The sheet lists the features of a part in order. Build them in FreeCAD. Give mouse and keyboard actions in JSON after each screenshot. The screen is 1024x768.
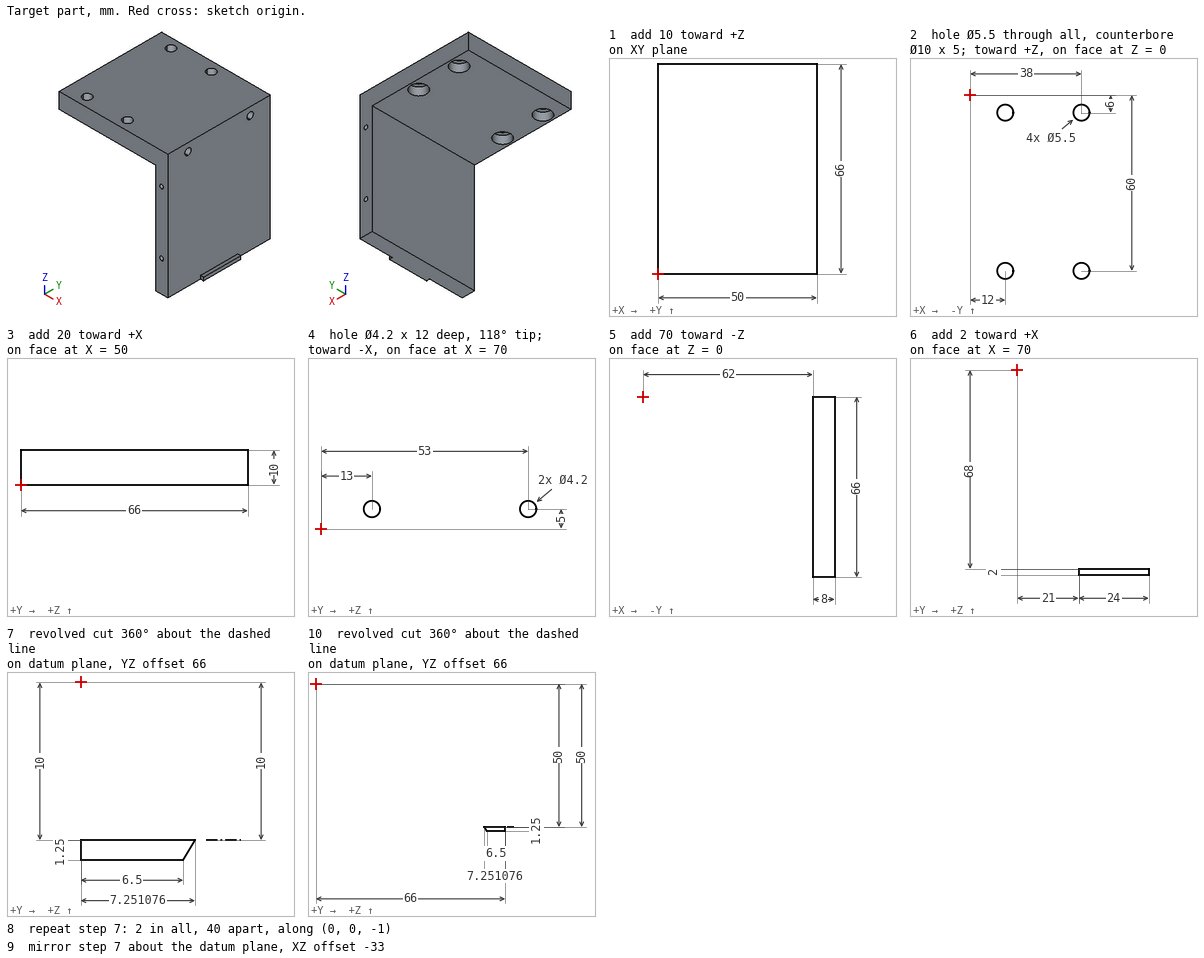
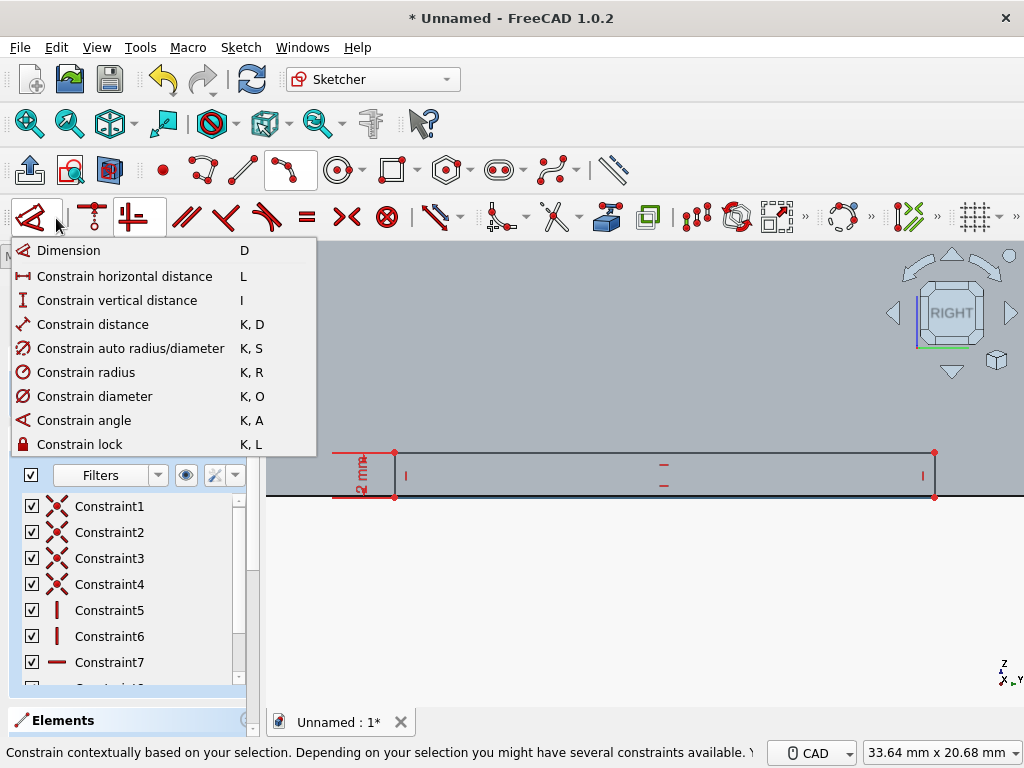
{"action": "left_click", "coordinate": [164, 276]}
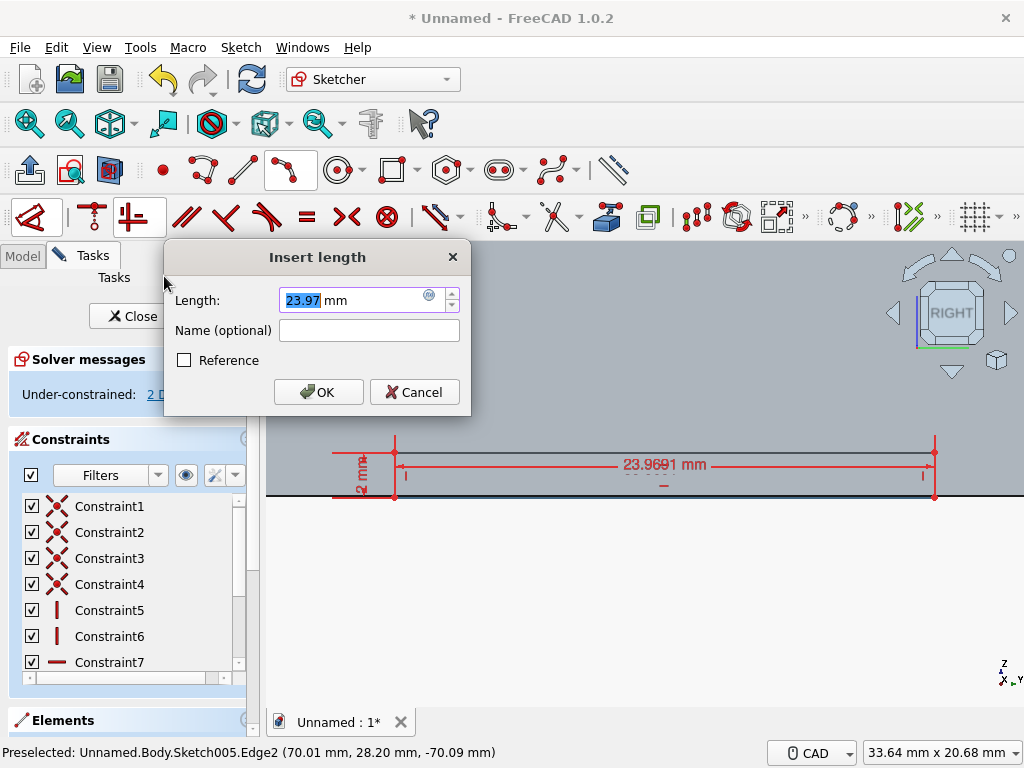
{"action": "type", "text": "24"}
{"action": "key", "text": "Return"}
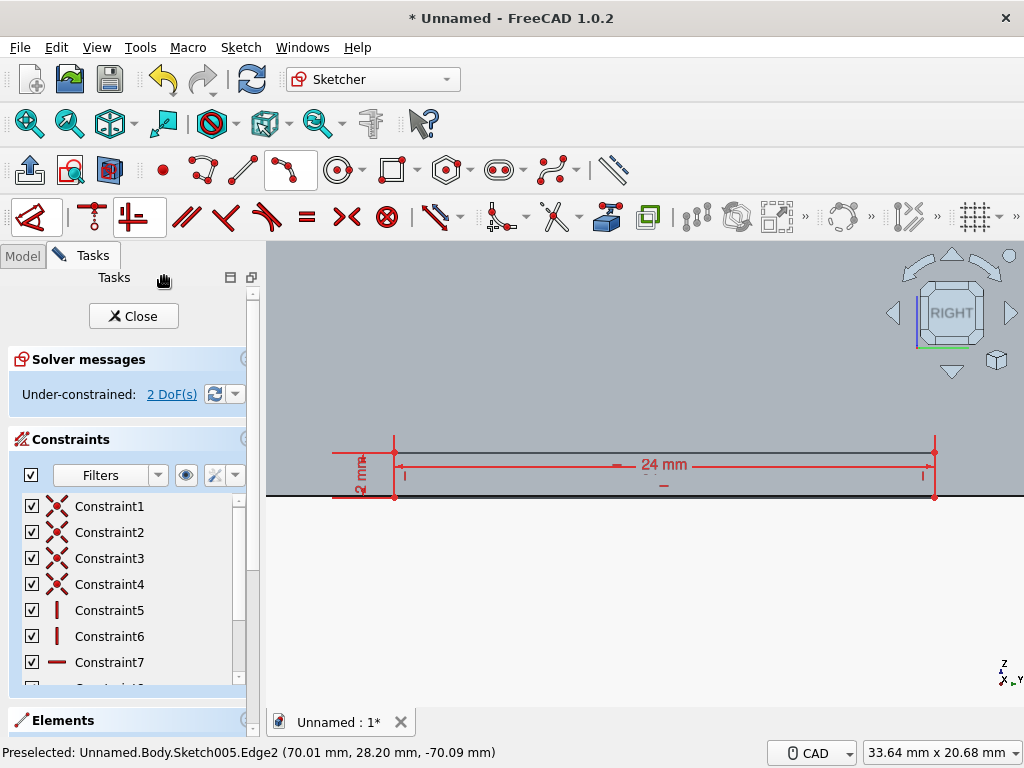
{"action": "left_click", "coordinate": [394, 453]}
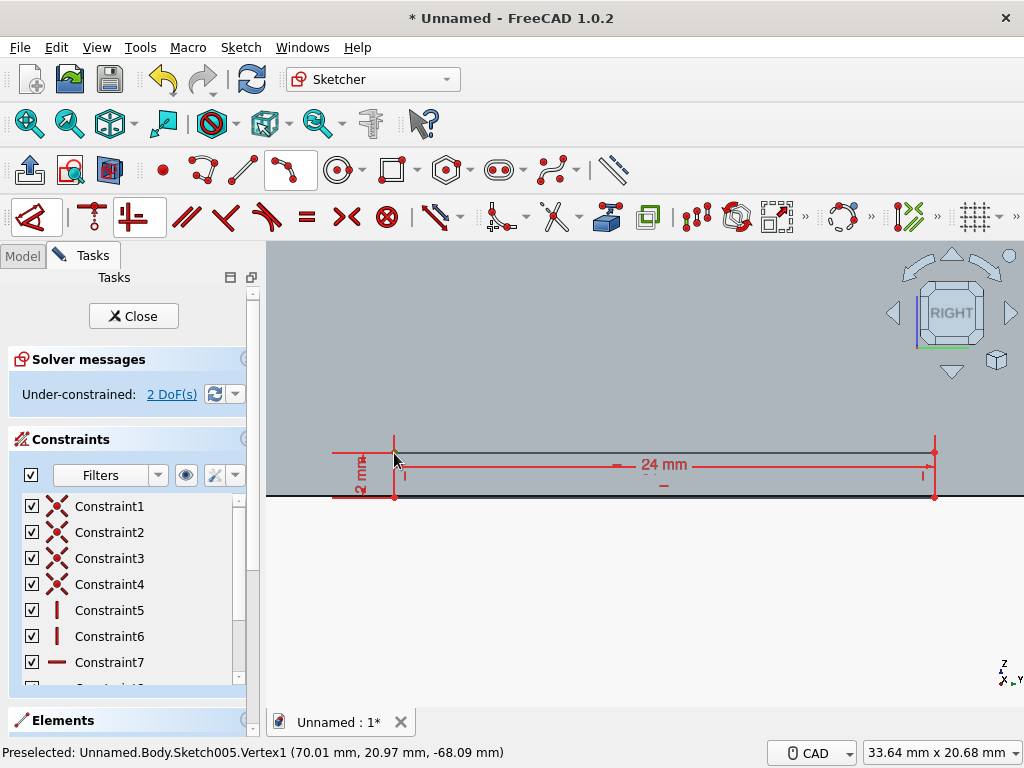
{"action": "key", "text": "l"}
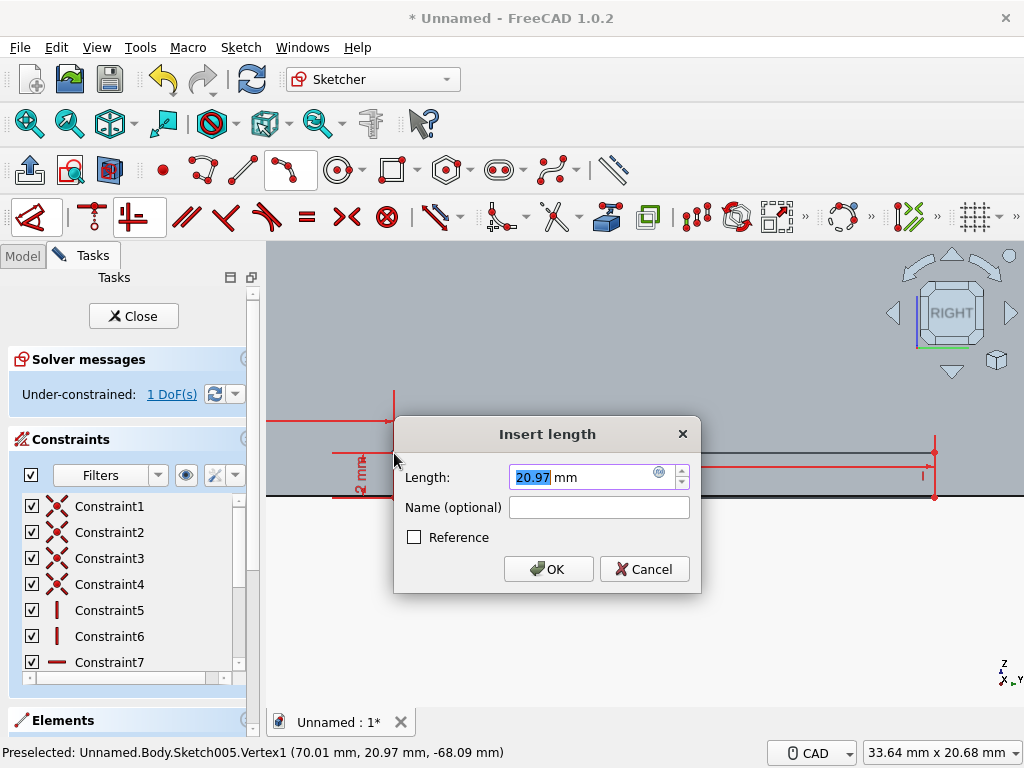
{"action": "type", "text": "21"}
{"action": "key", "text": "Return"}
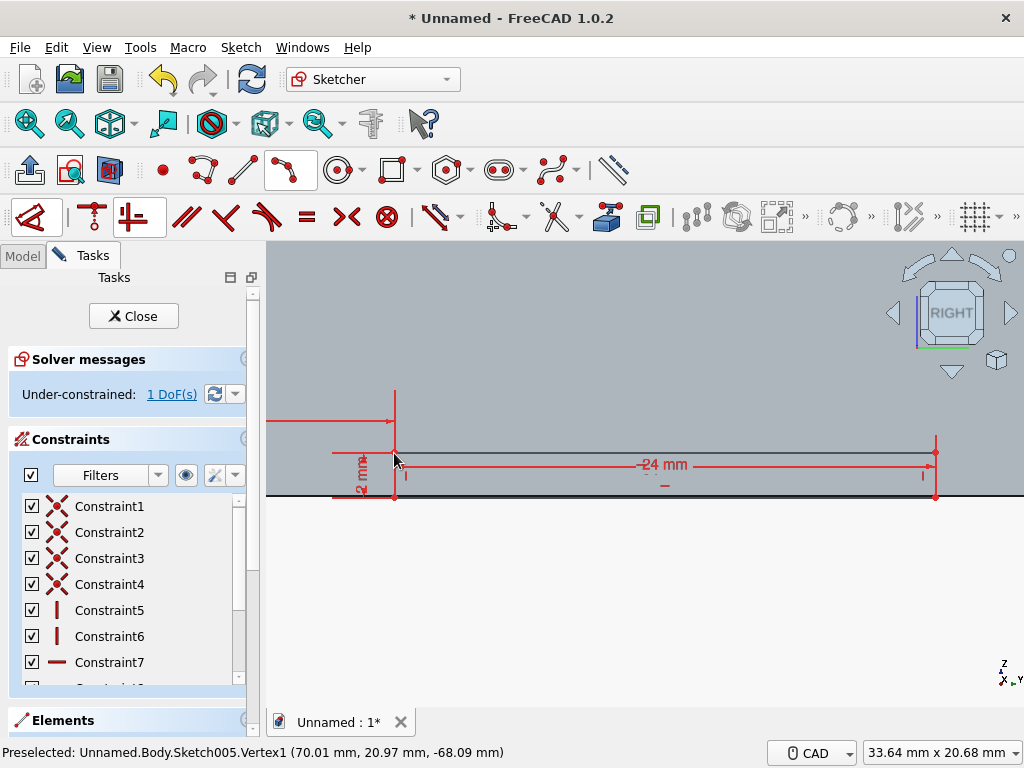
{"action": "left_click", "coordinate": [395, 453]}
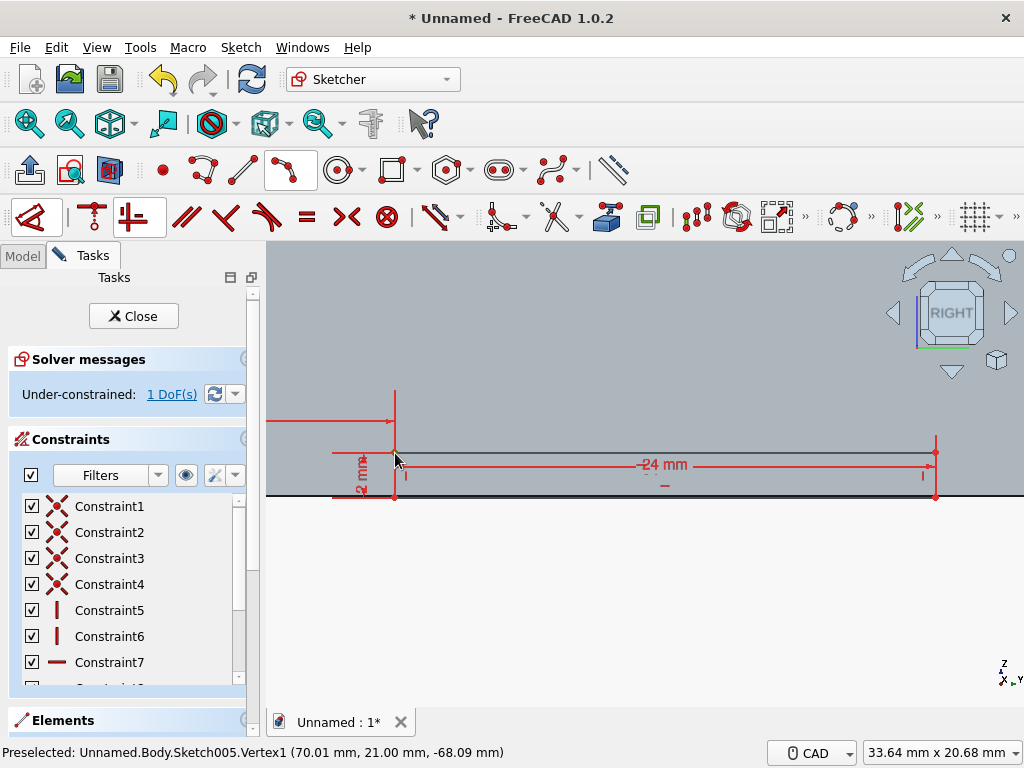
{"action": "left_click", "coordinate": [56, 218]}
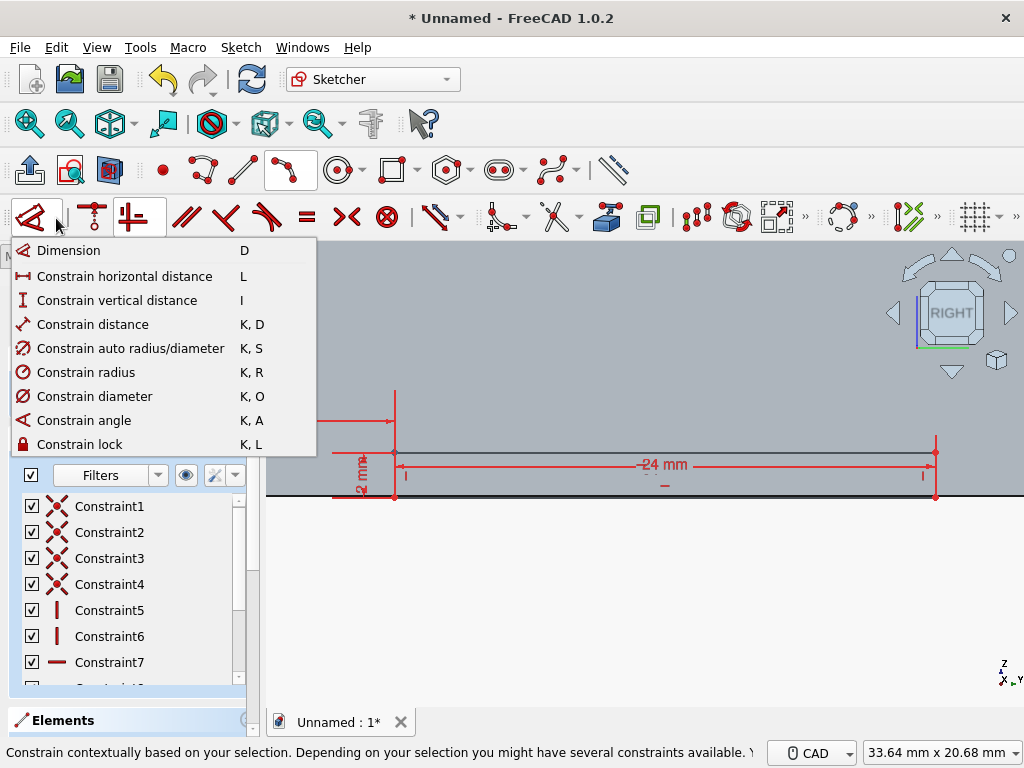
{"action": "left_click", "coordinate": [164, 300]}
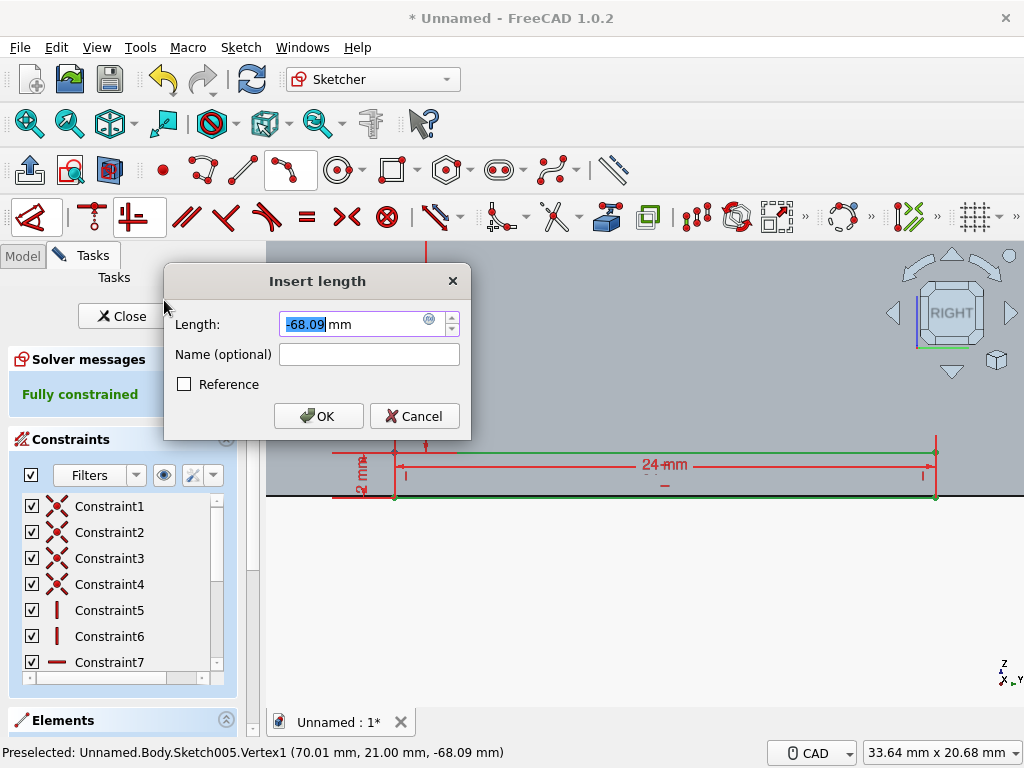
{"action": "type", "text": "-68"}
{"action": "key", "text": "Return"}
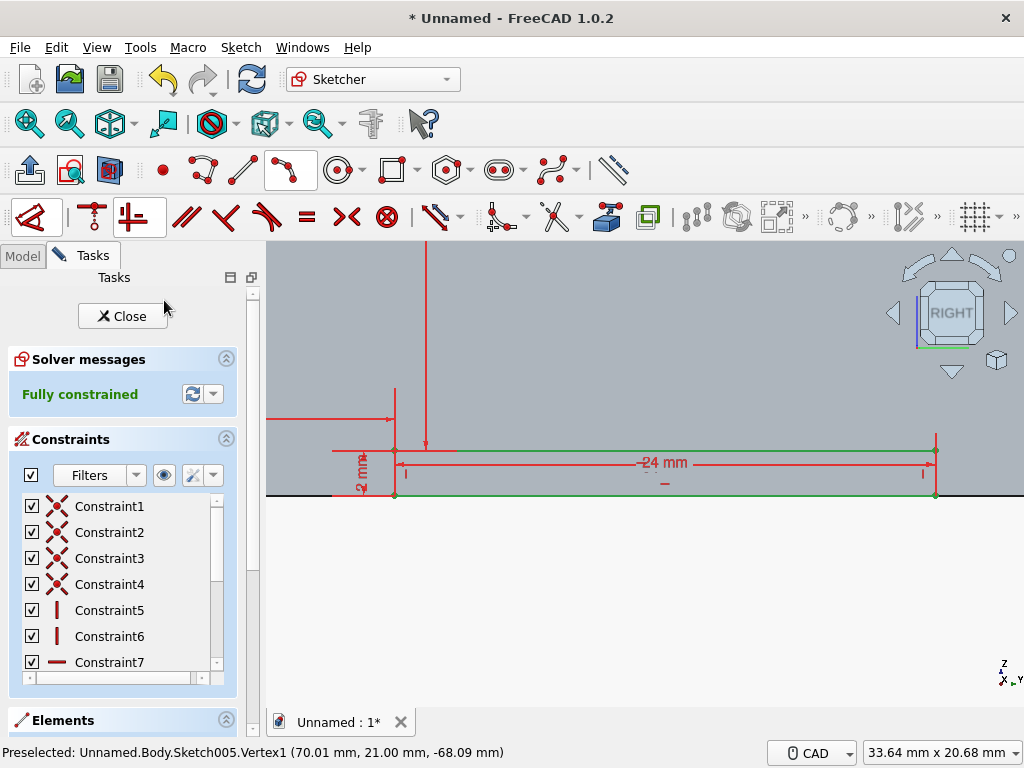
{"action": "left_click", "coordinate": [123, 316]}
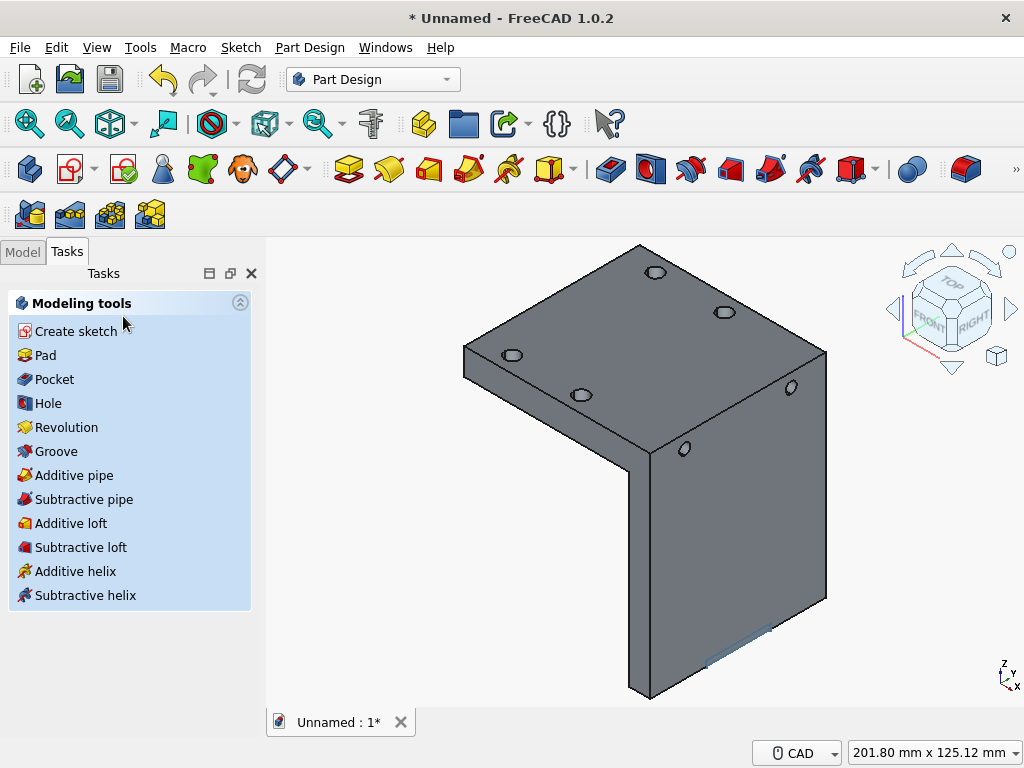
{"action": "left_click", "coordinate": [350, 170]}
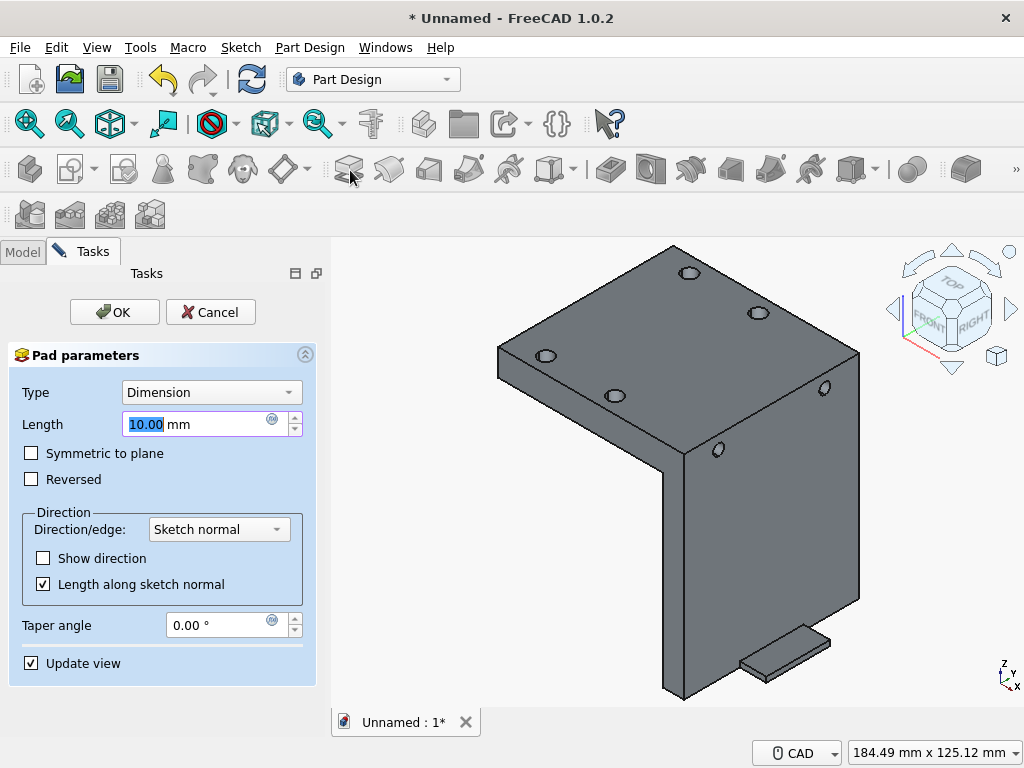
{"action": "type", "text": "2"}
{"action": "key", "text": "Tab"}